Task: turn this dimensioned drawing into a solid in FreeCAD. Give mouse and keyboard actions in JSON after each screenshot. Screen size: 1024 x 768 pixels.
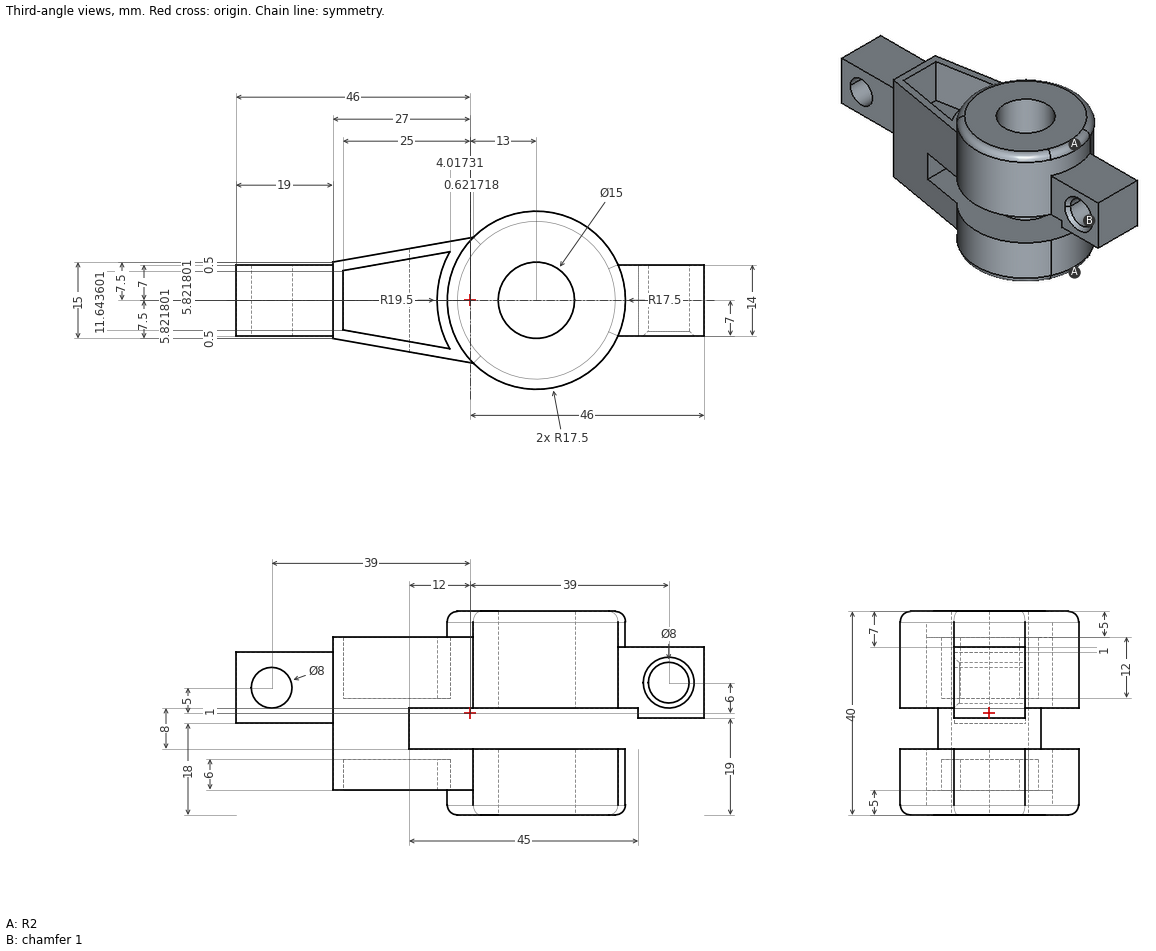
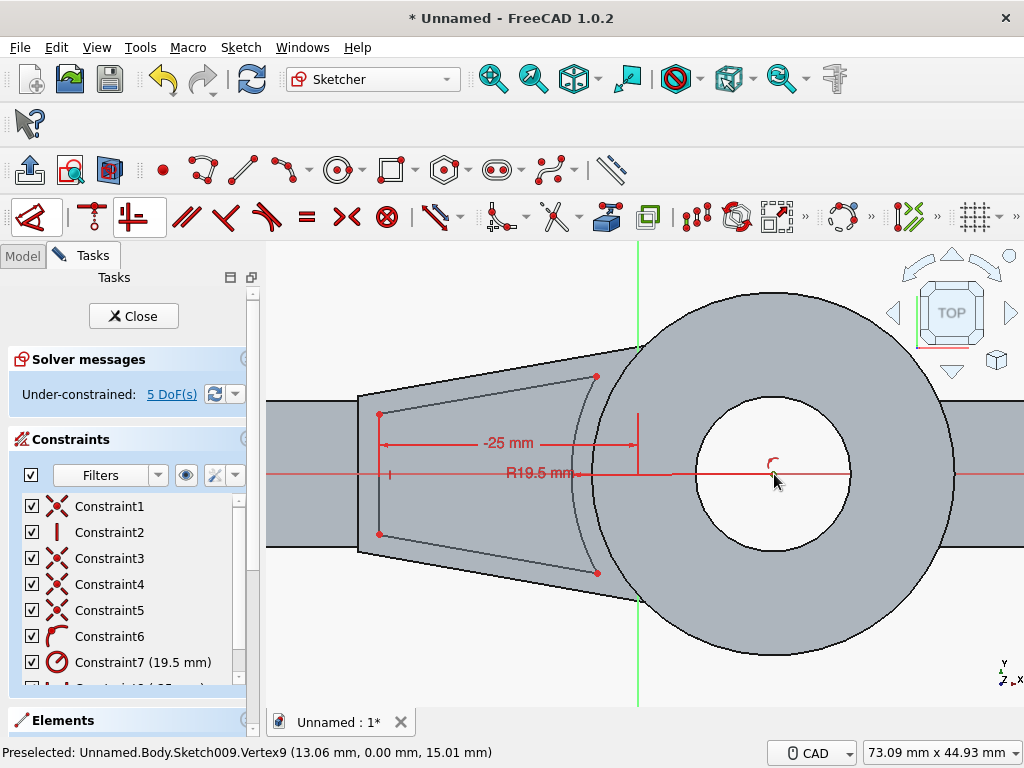
{"action": "left_click", "coordinate": [56, 218]}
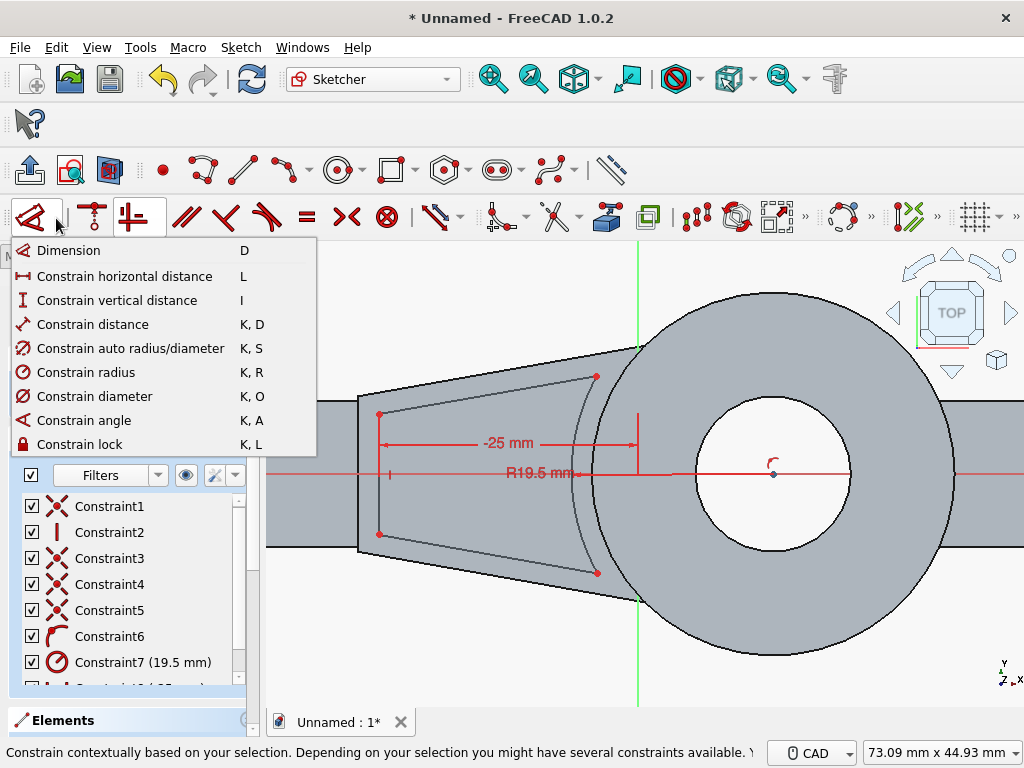
{"action": "left_click", "coordinate": [164, 276]}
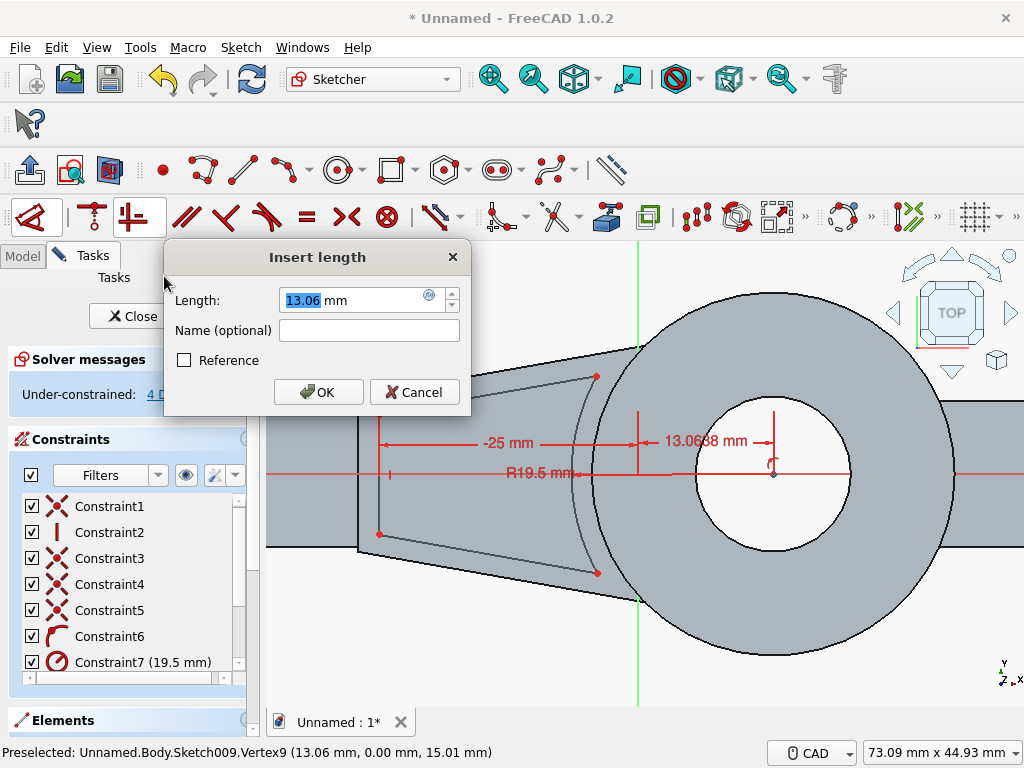
{"action": "type", "text": "13"}
{"action": "key", "text": "Return"}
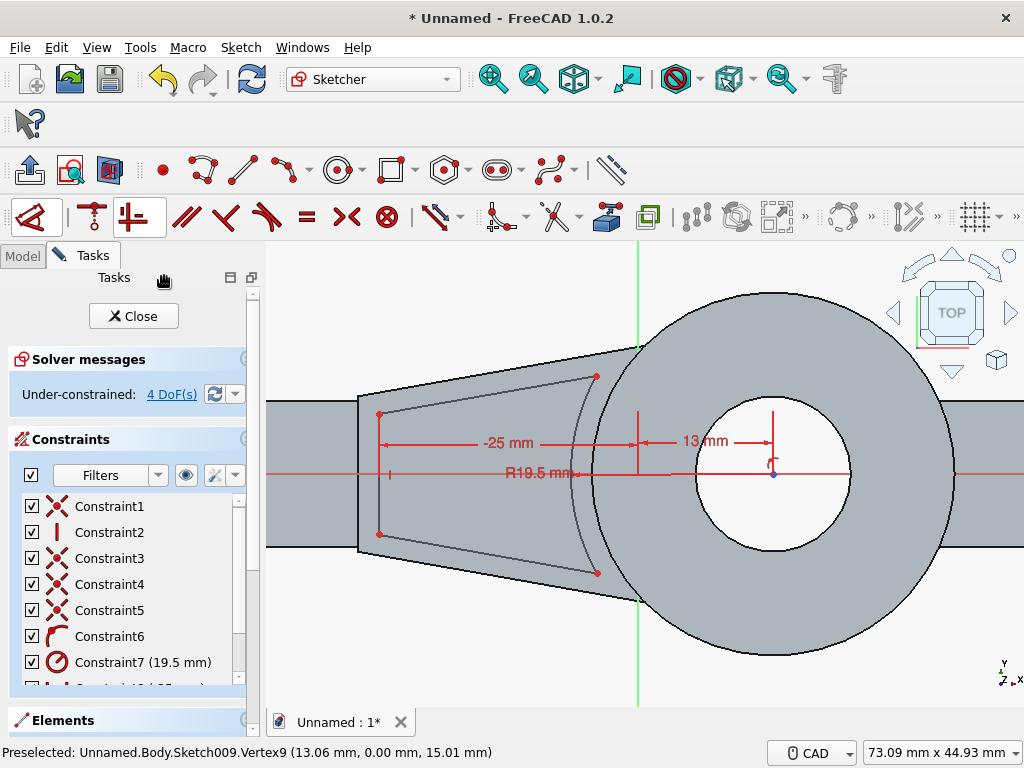
{"action": "left_click", "coordinate": [596, 376]}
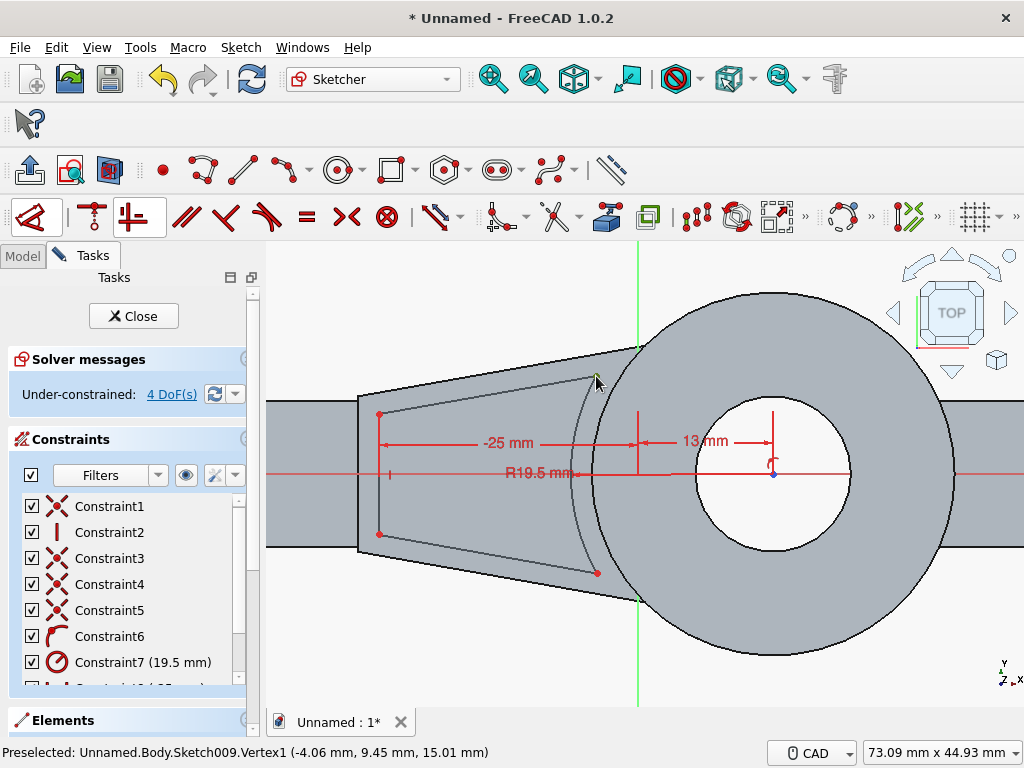
{"action": "left_click", "coordinate": [56, 218]}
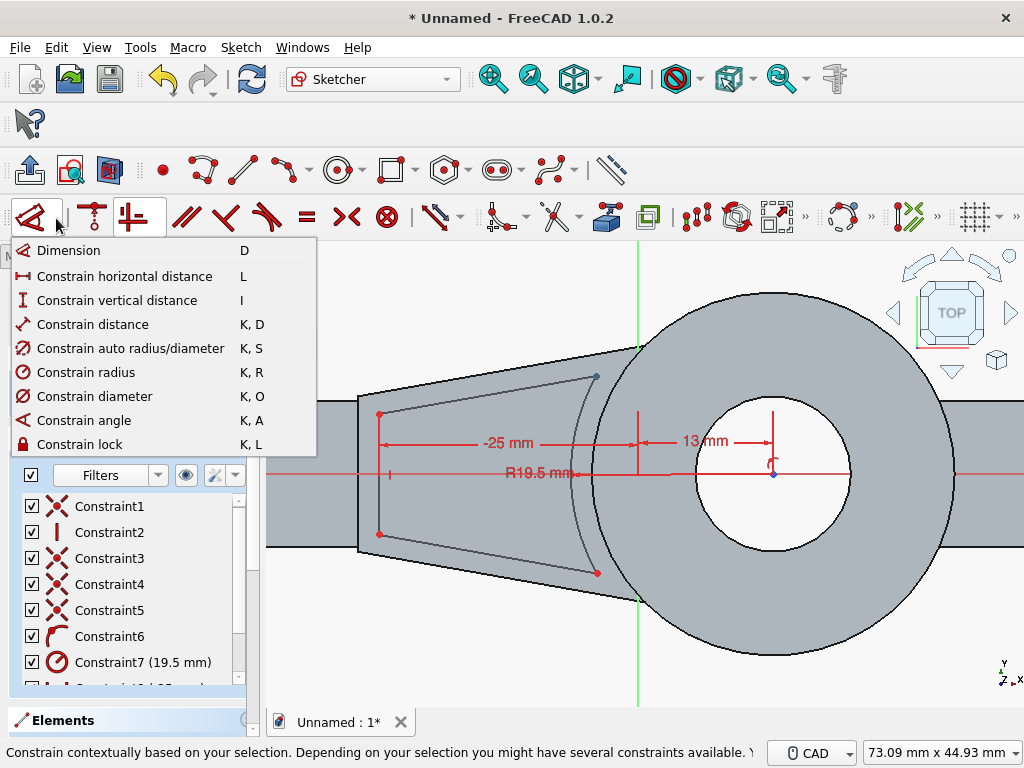
{"action": "left_click", "coordinate": [164, 276]}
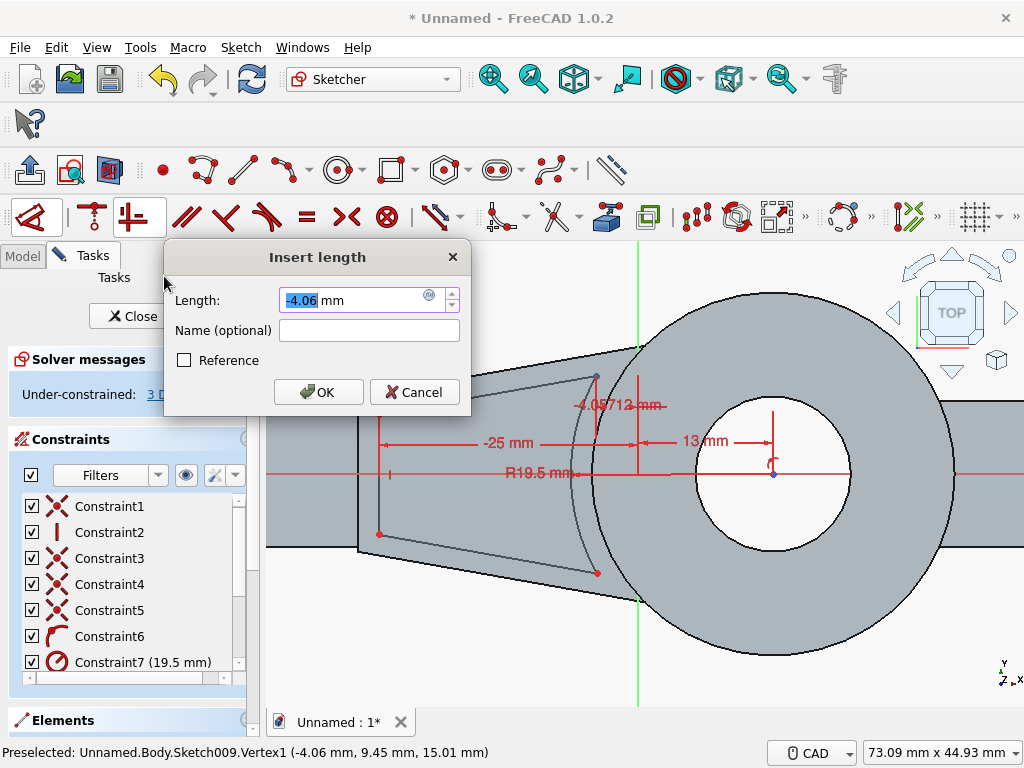
{"action": "type", "text": "-4.01731"}
{"action": "key", "text": "Return"}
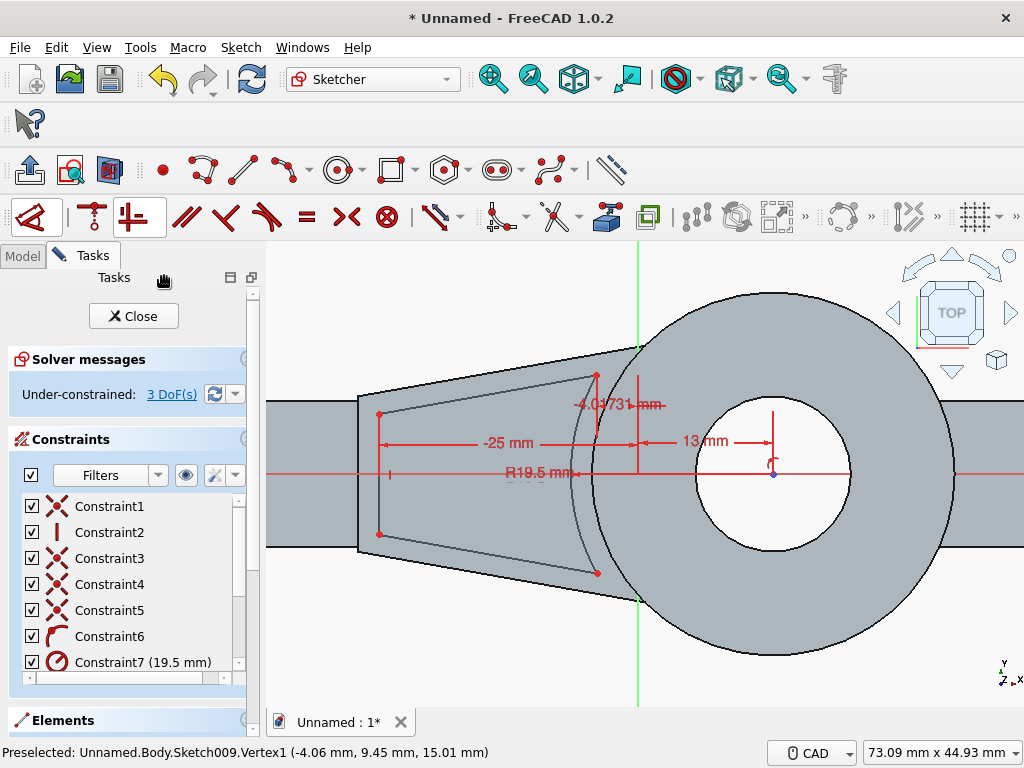
{"action": "left_click", "coordinate": [597, 574]}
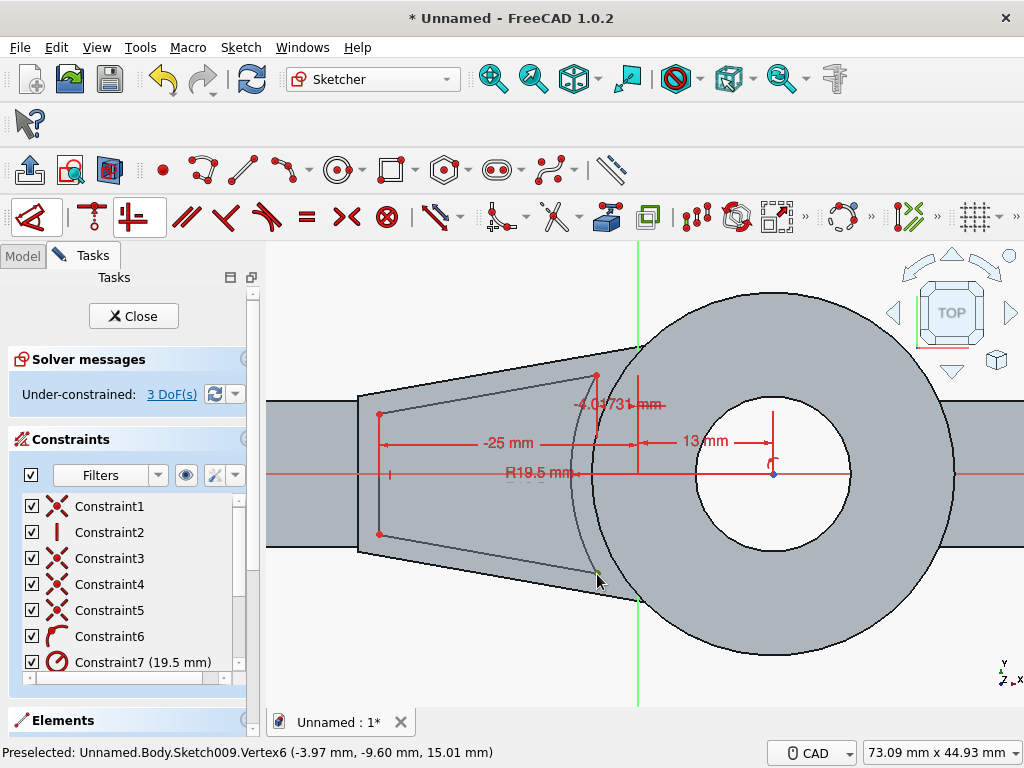
{"action": "left_click", "coordinate": [56, 218]}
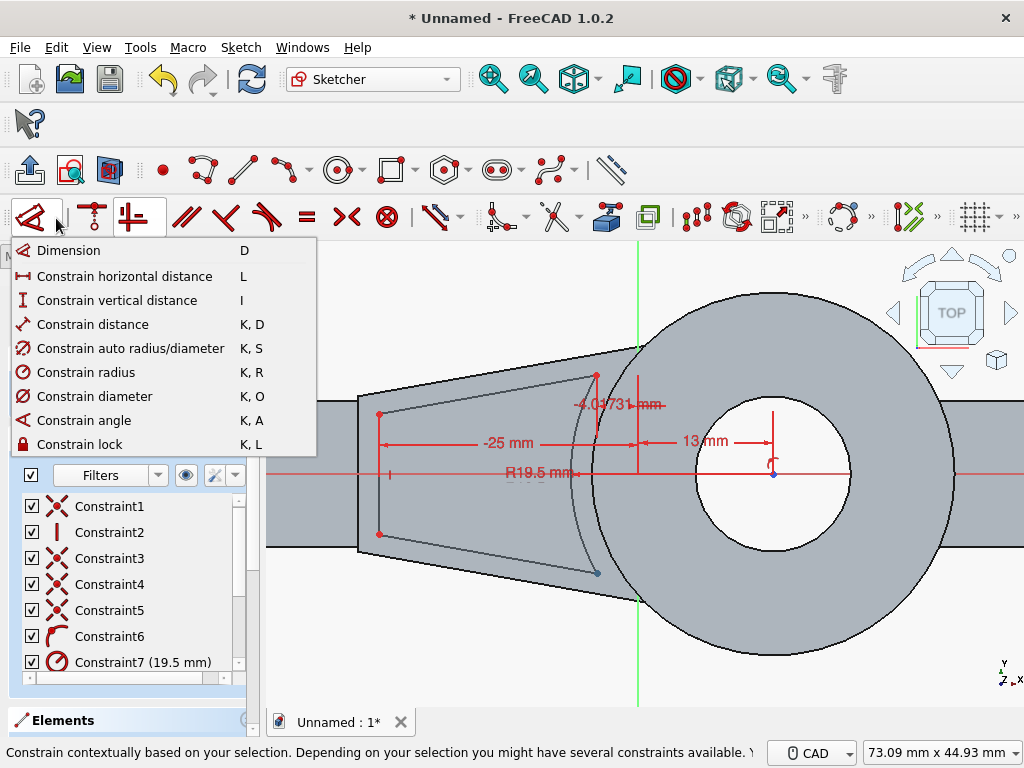
{"action": "left_click", "coordinate": [164, 276]}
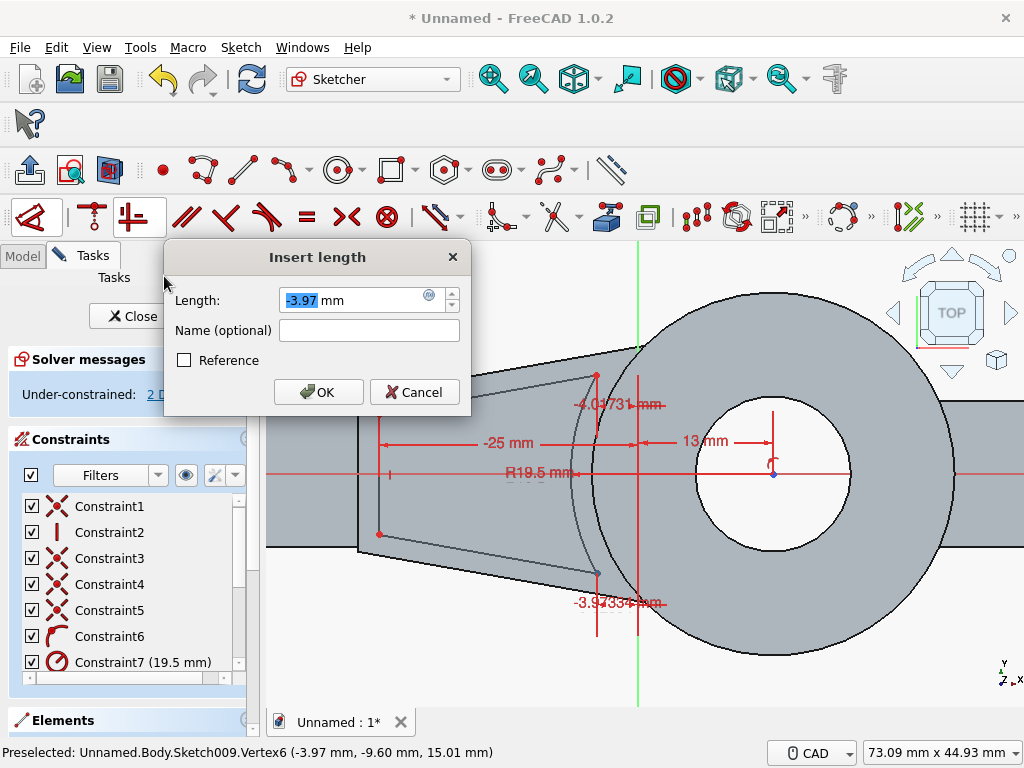
{"action": "type", "text": "-4.01731"}
{"action": "key", "text": "Return"}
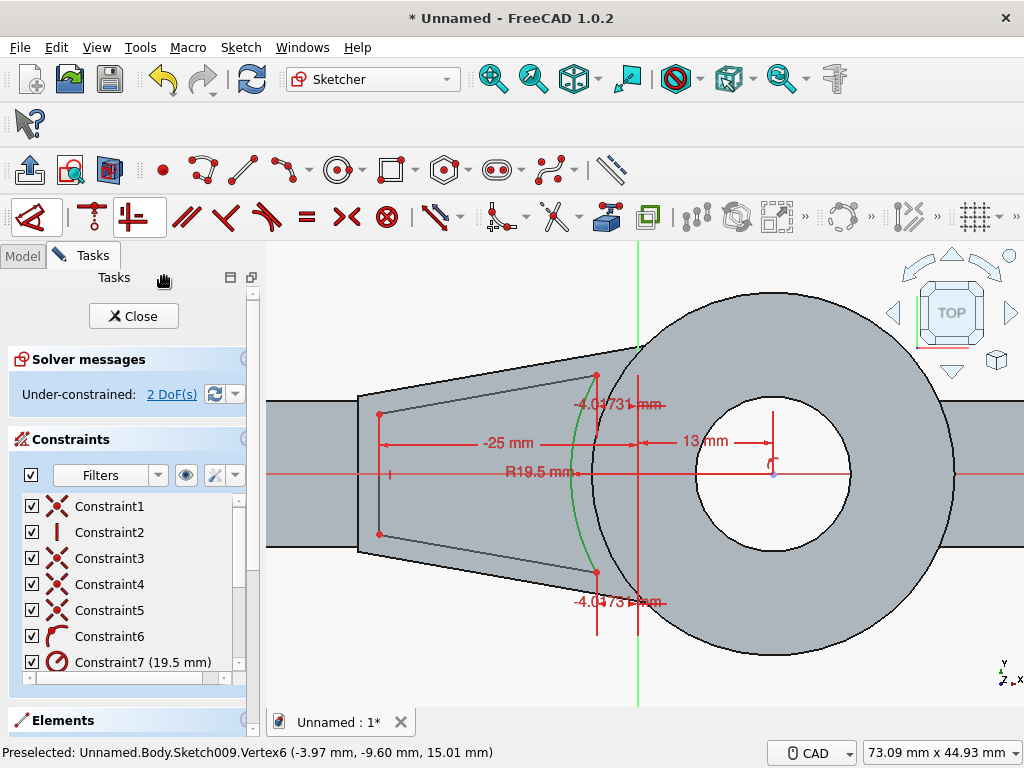
{"action": "left_click", "coordinate": [379, 450]}